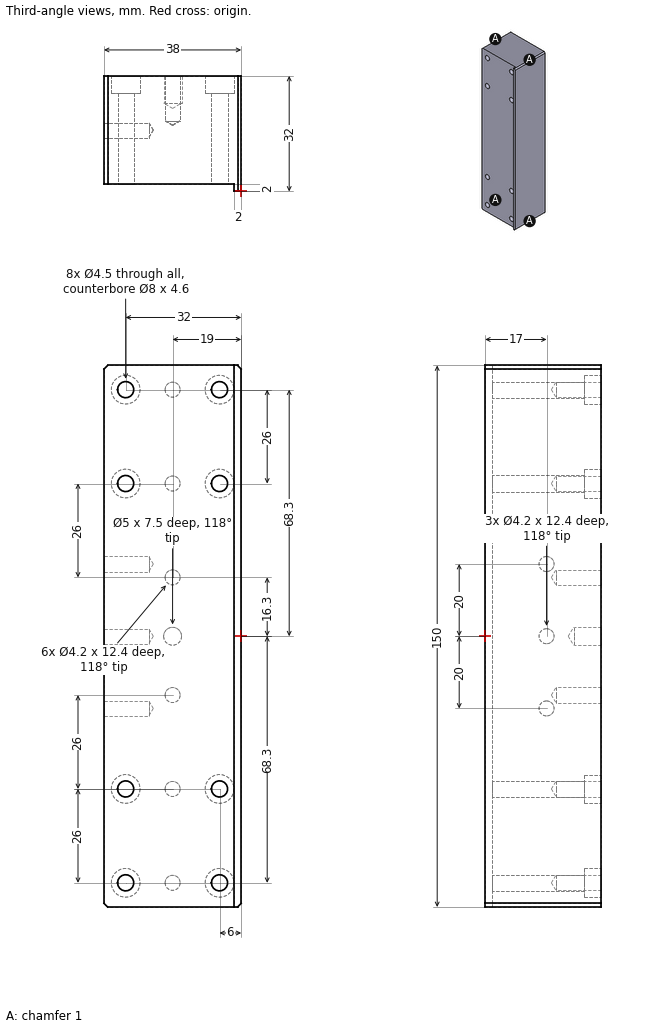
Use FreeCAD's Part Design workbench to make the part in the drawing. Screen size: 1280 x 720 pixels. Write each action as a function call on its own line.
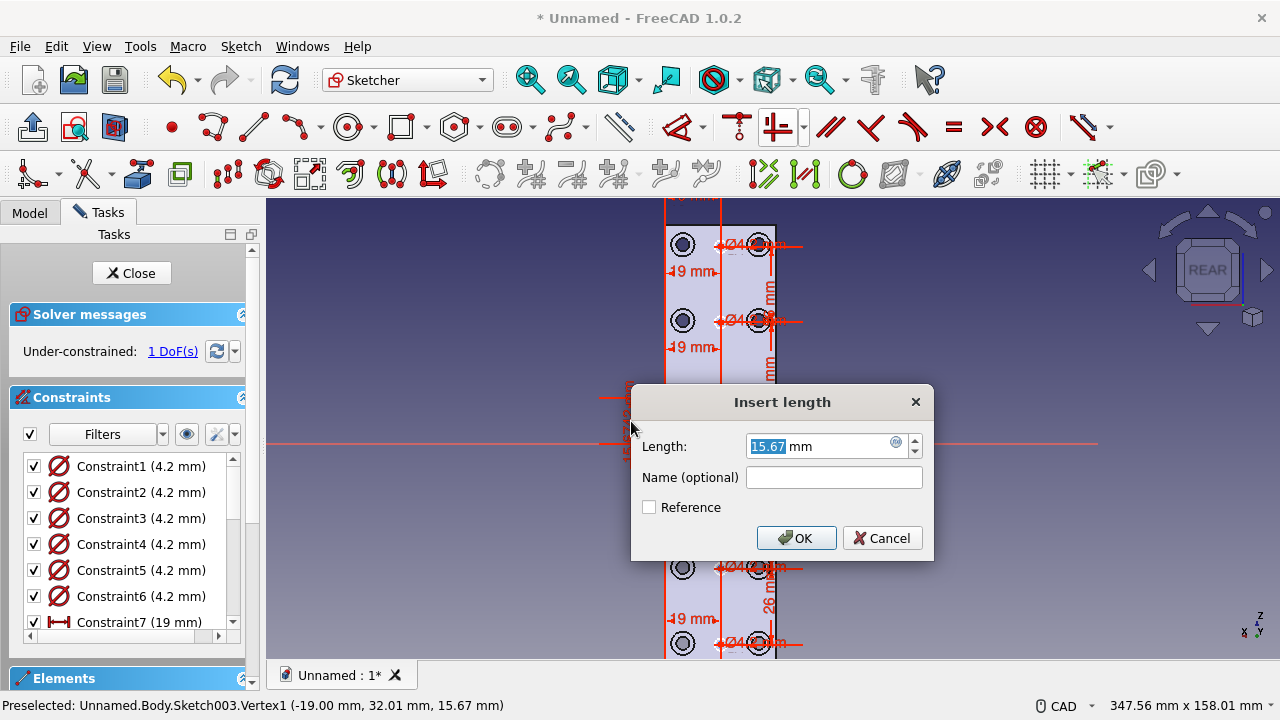
text(16.3)
key(Return)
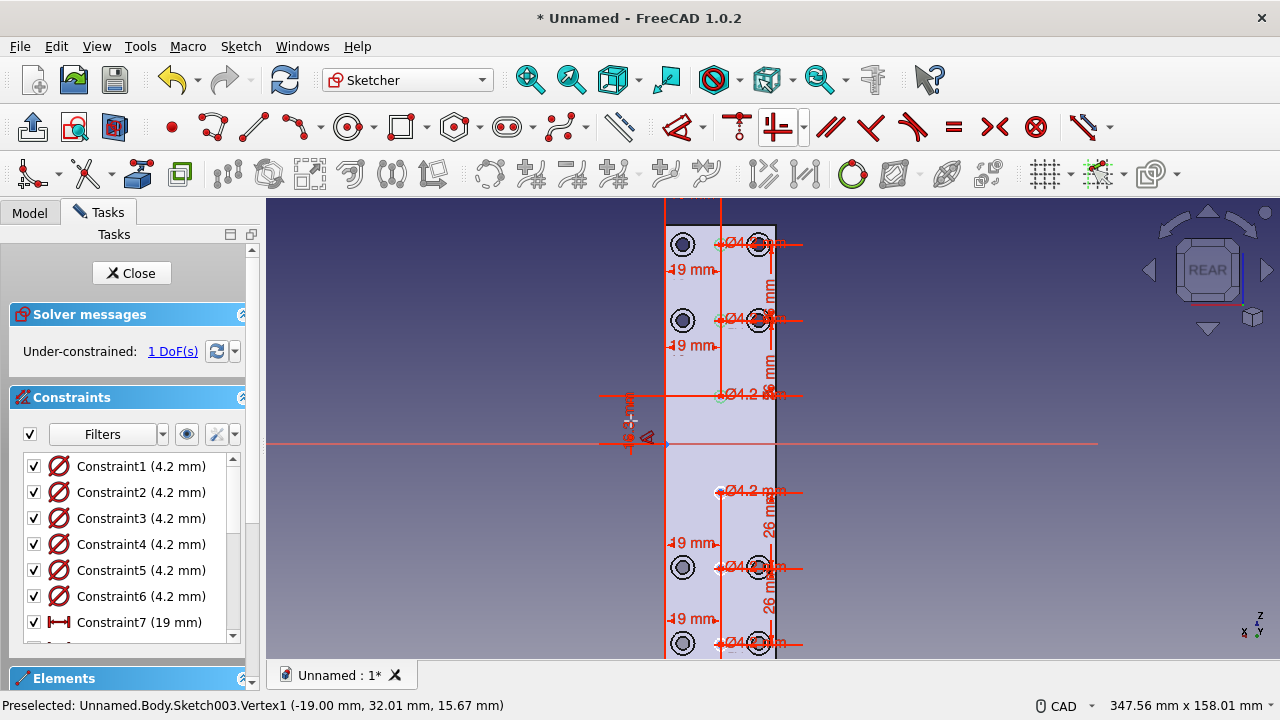
scroll(721, 397, down, 2)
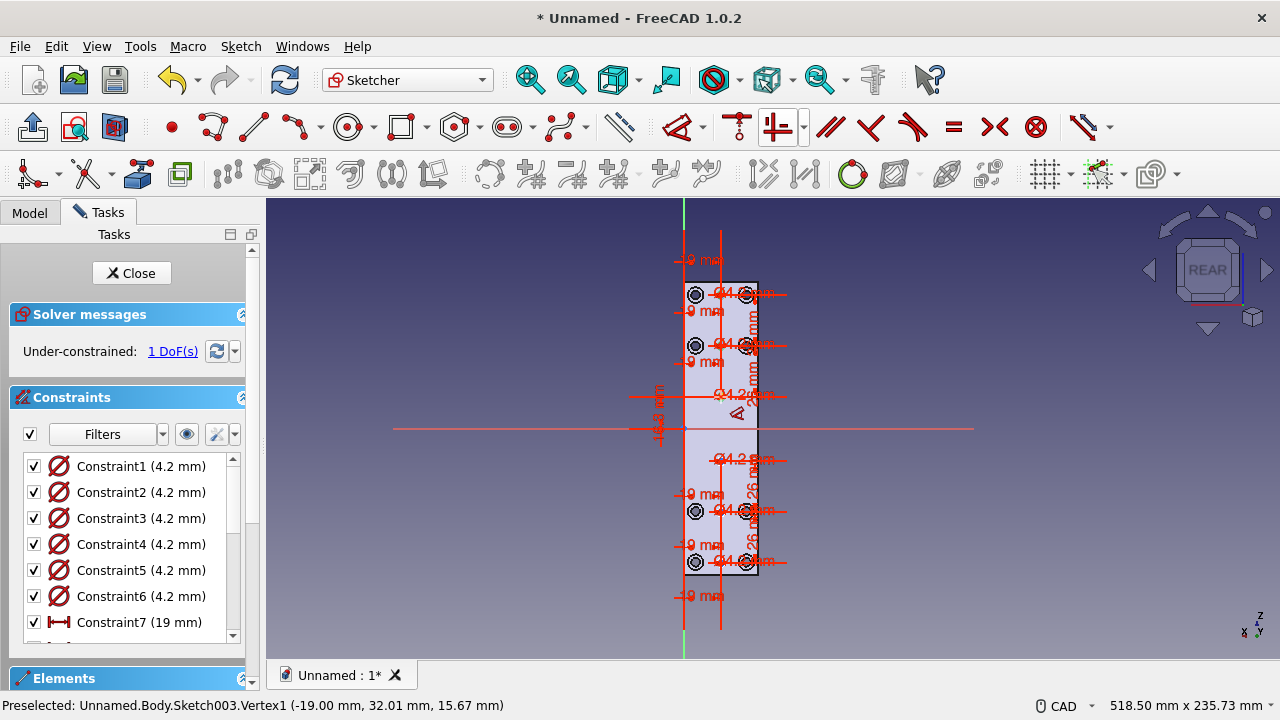
click(721, 563)
click(650, 465)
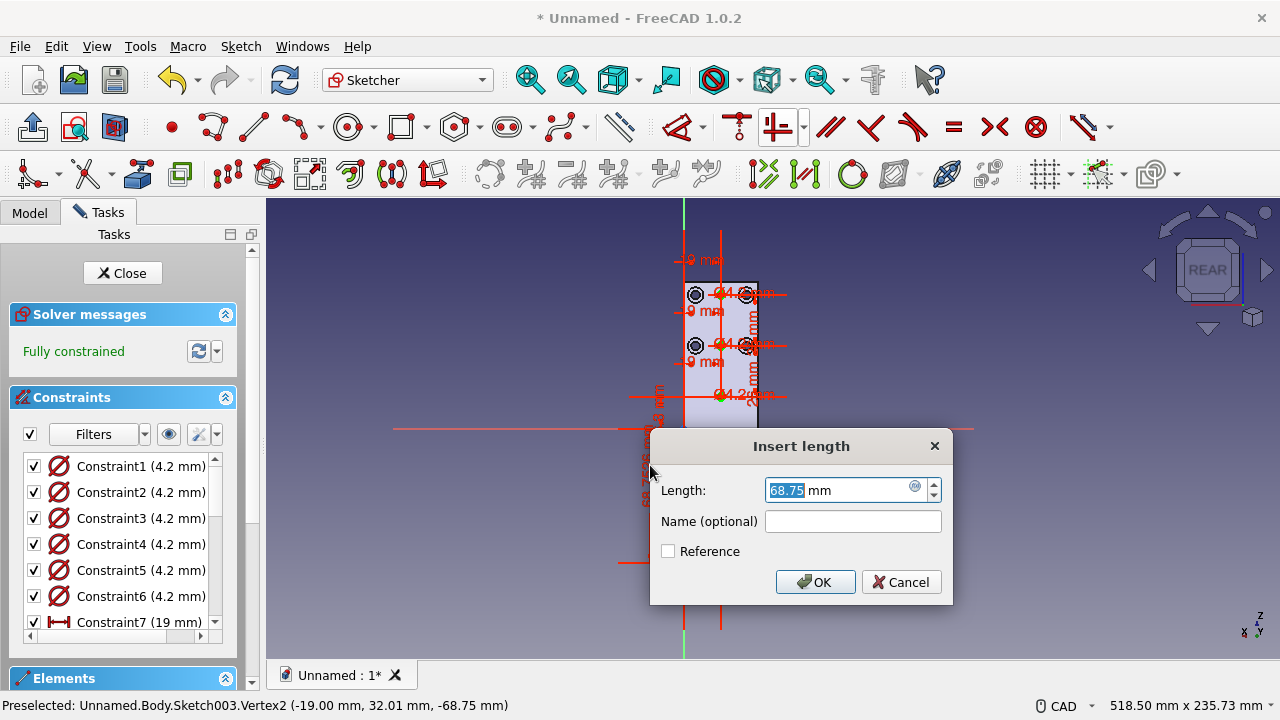
text(68.3)
key(Return)
key(Escape)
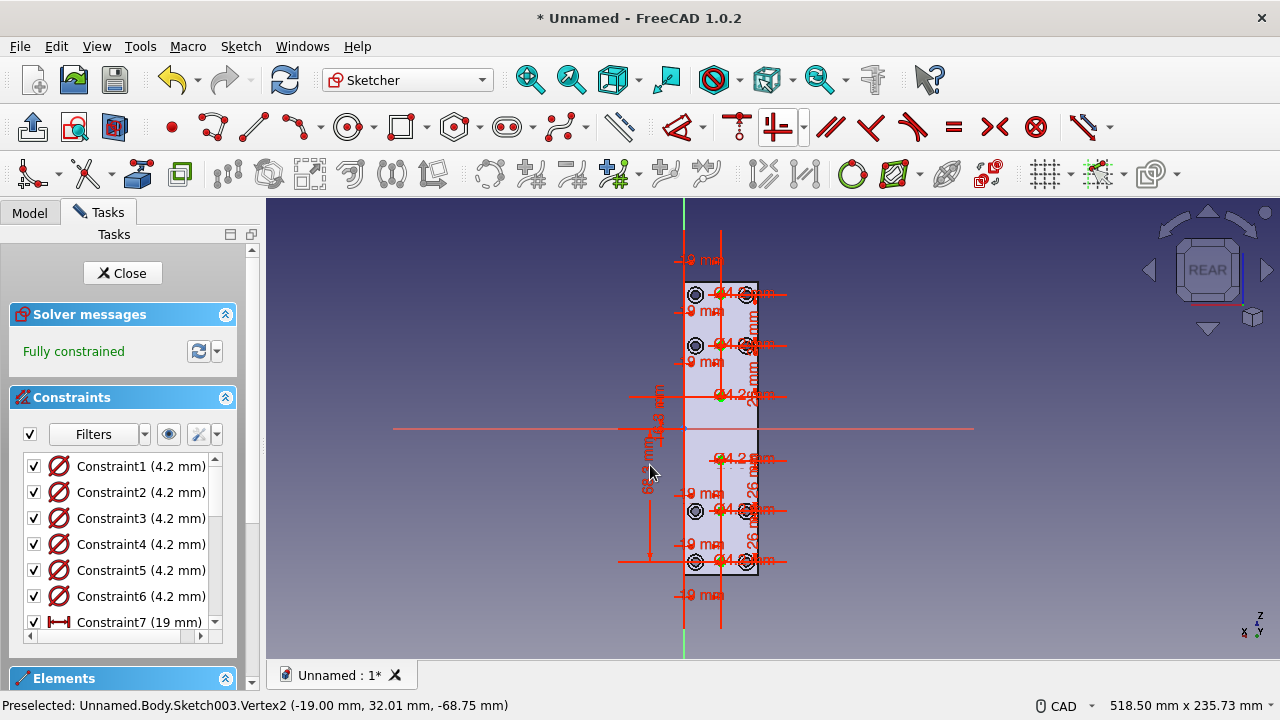
click(123, 273)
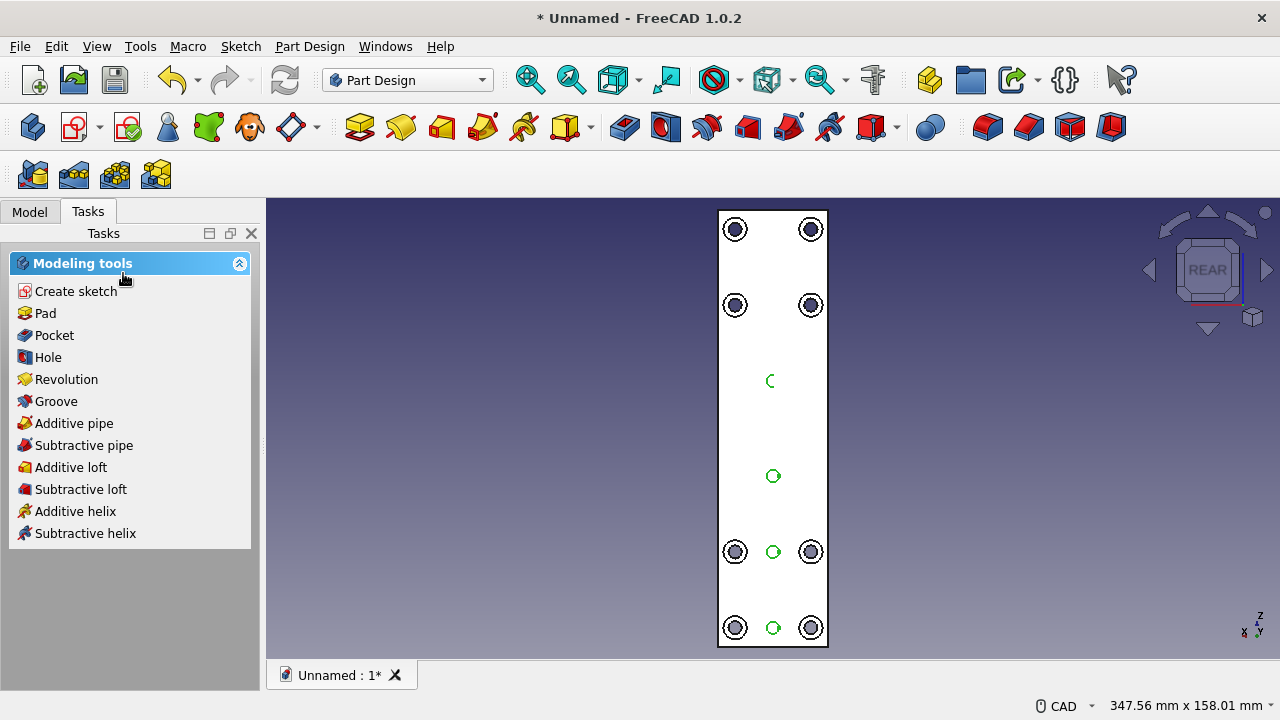
click(666, 128)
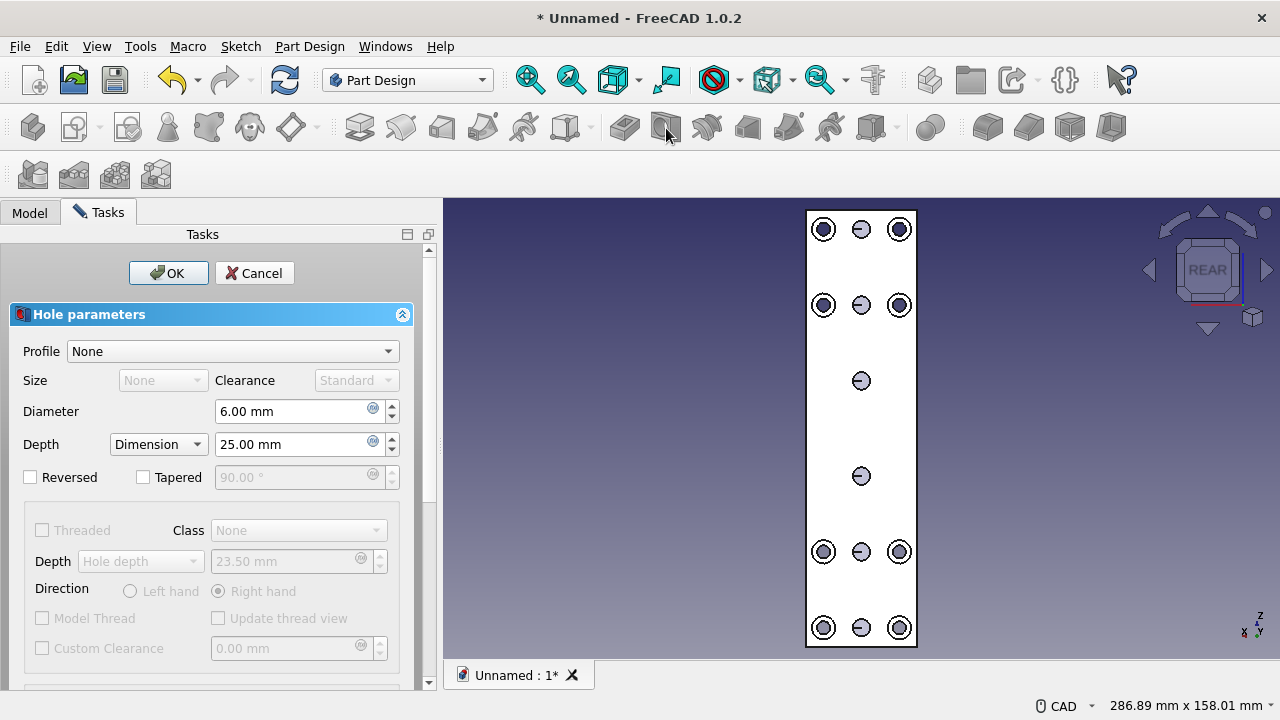
triple_click(300, 412)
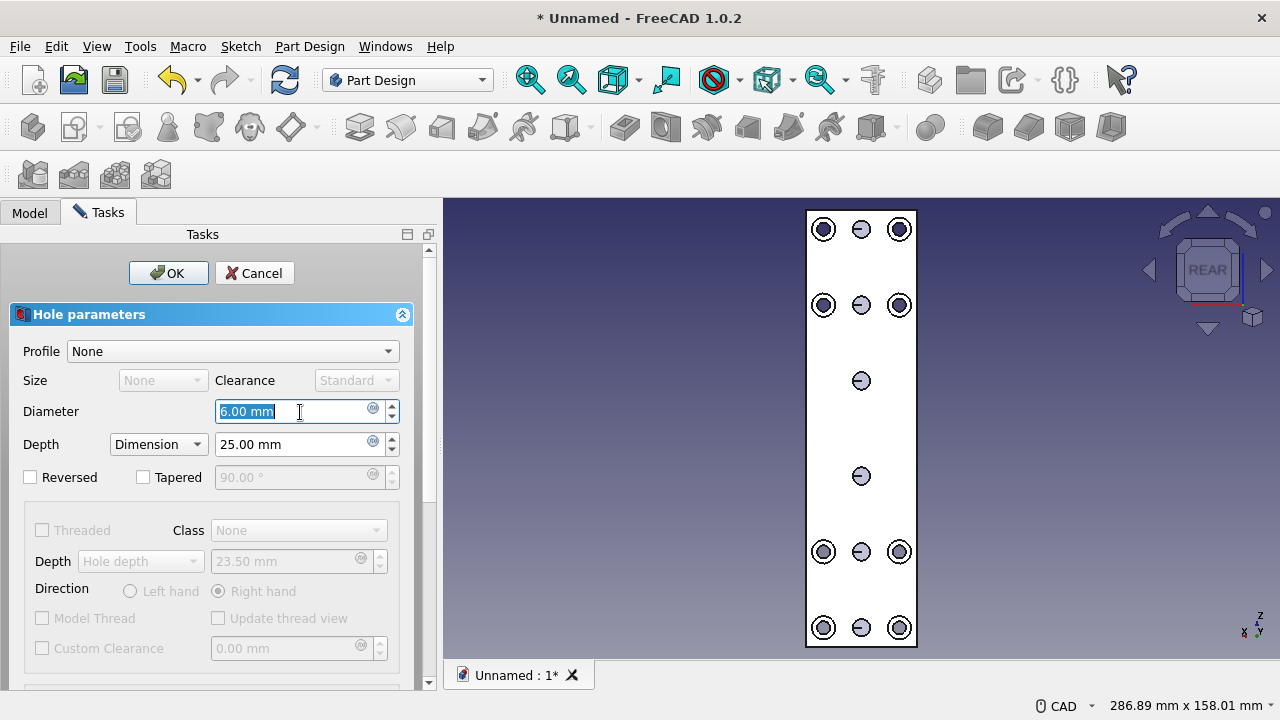
text(4.2)
key(Tab)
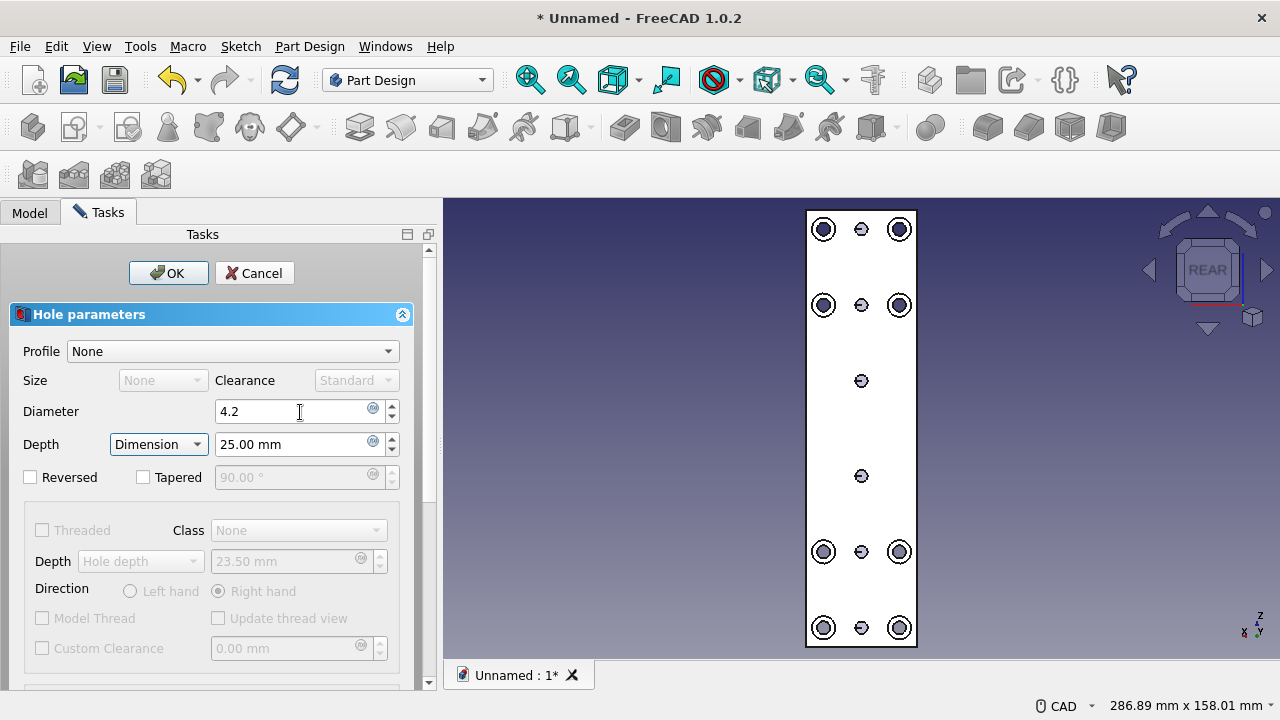
triple_click(300, 444)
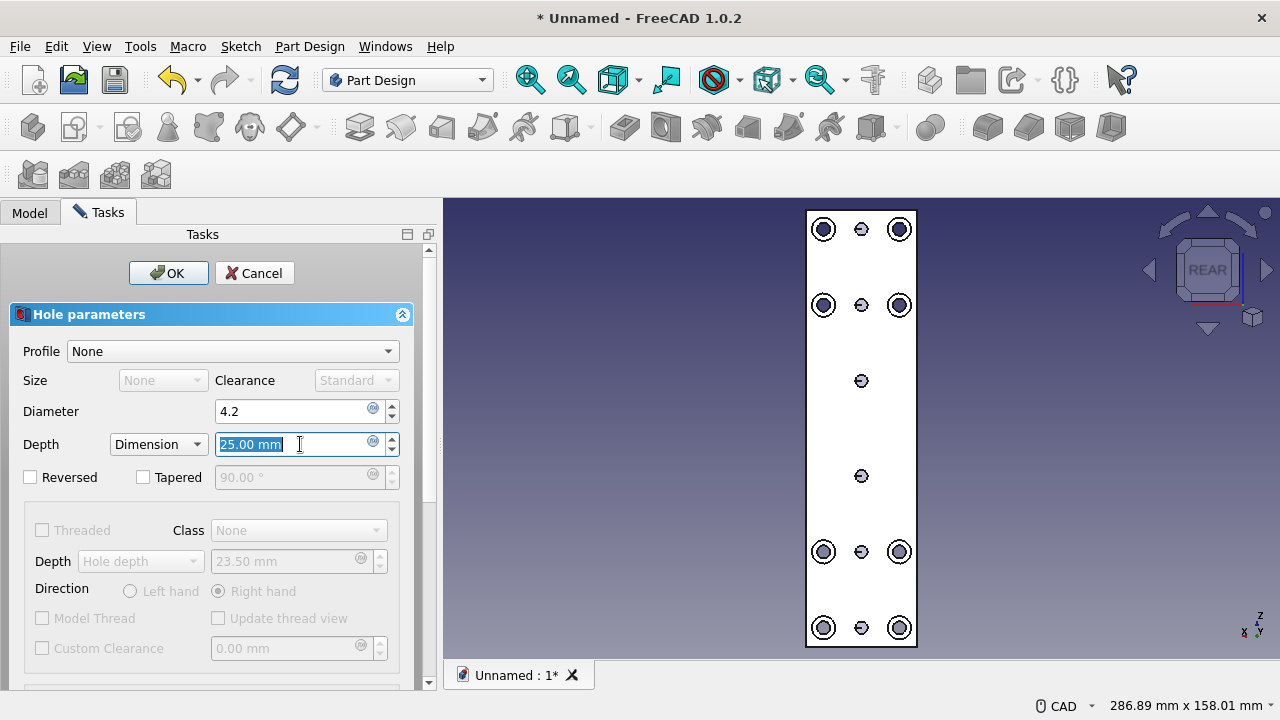
text(12.4)
key(Tab)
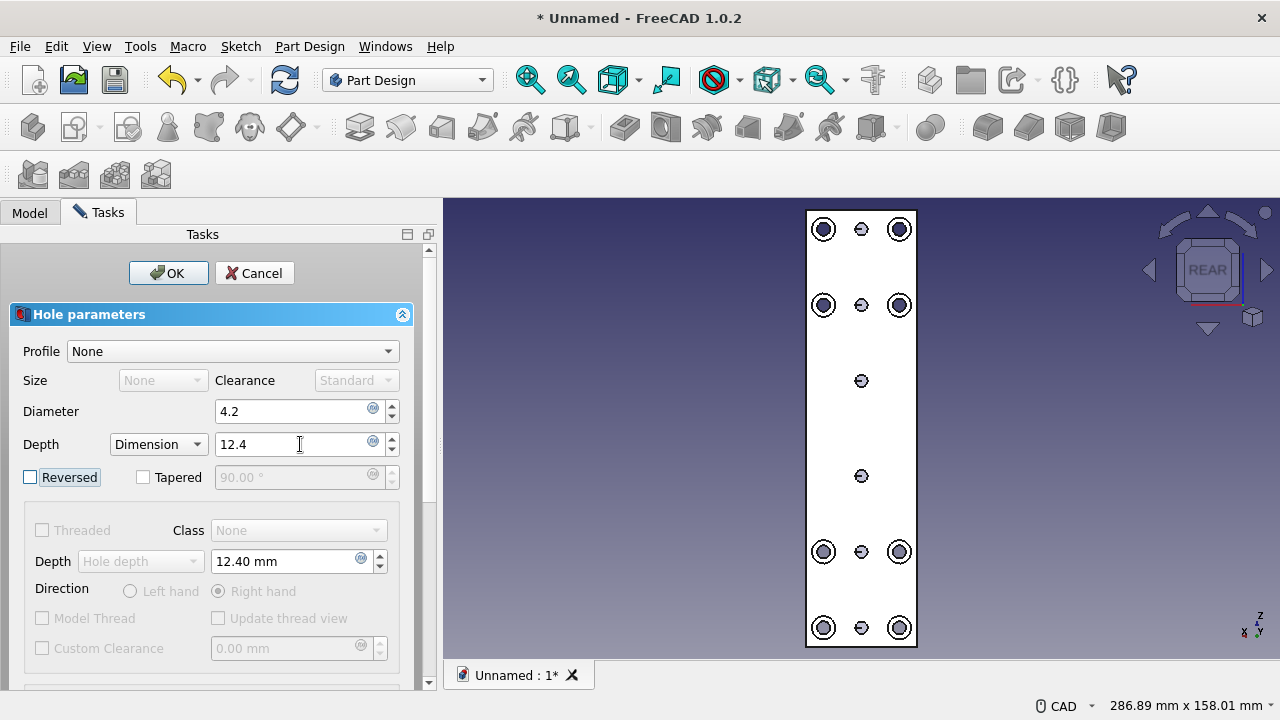
click(169, 273)